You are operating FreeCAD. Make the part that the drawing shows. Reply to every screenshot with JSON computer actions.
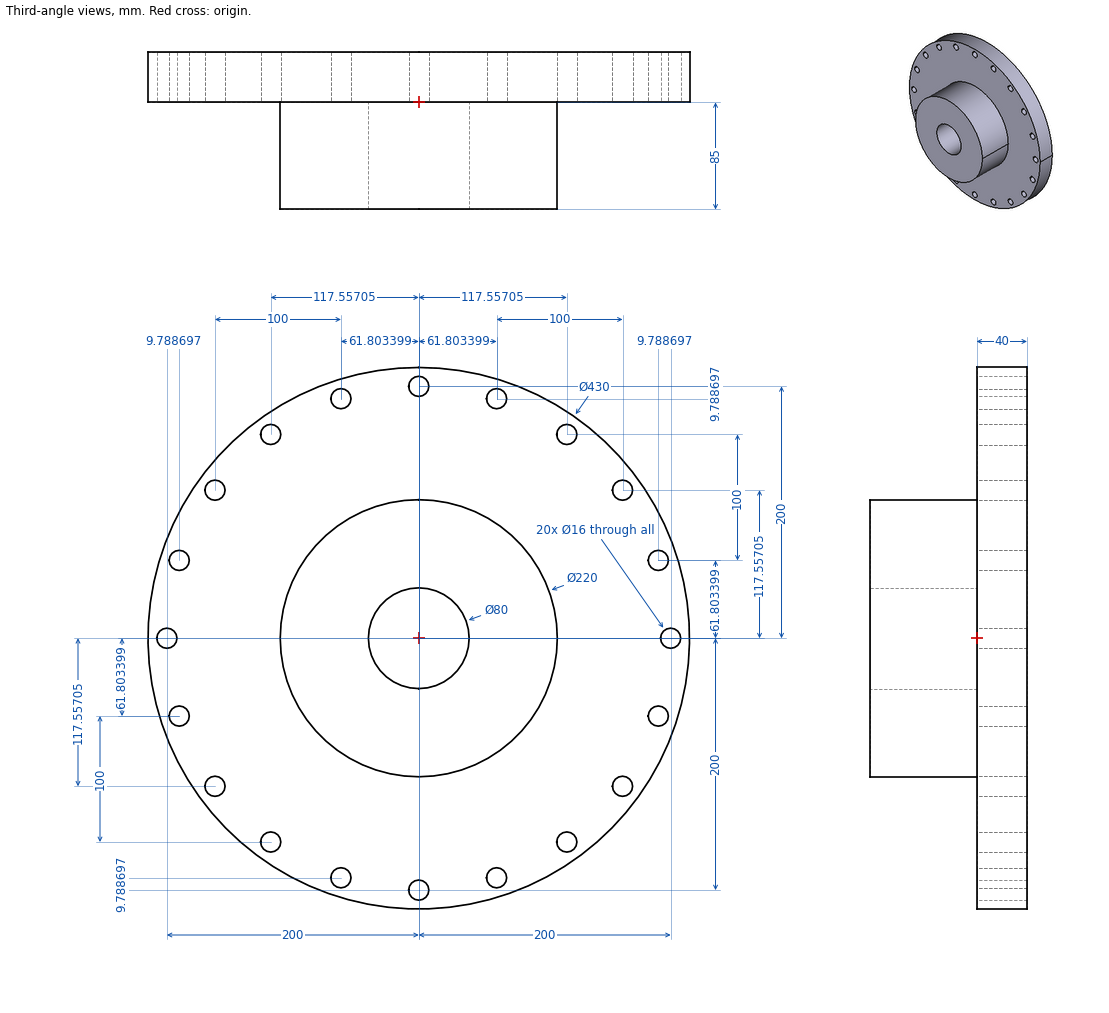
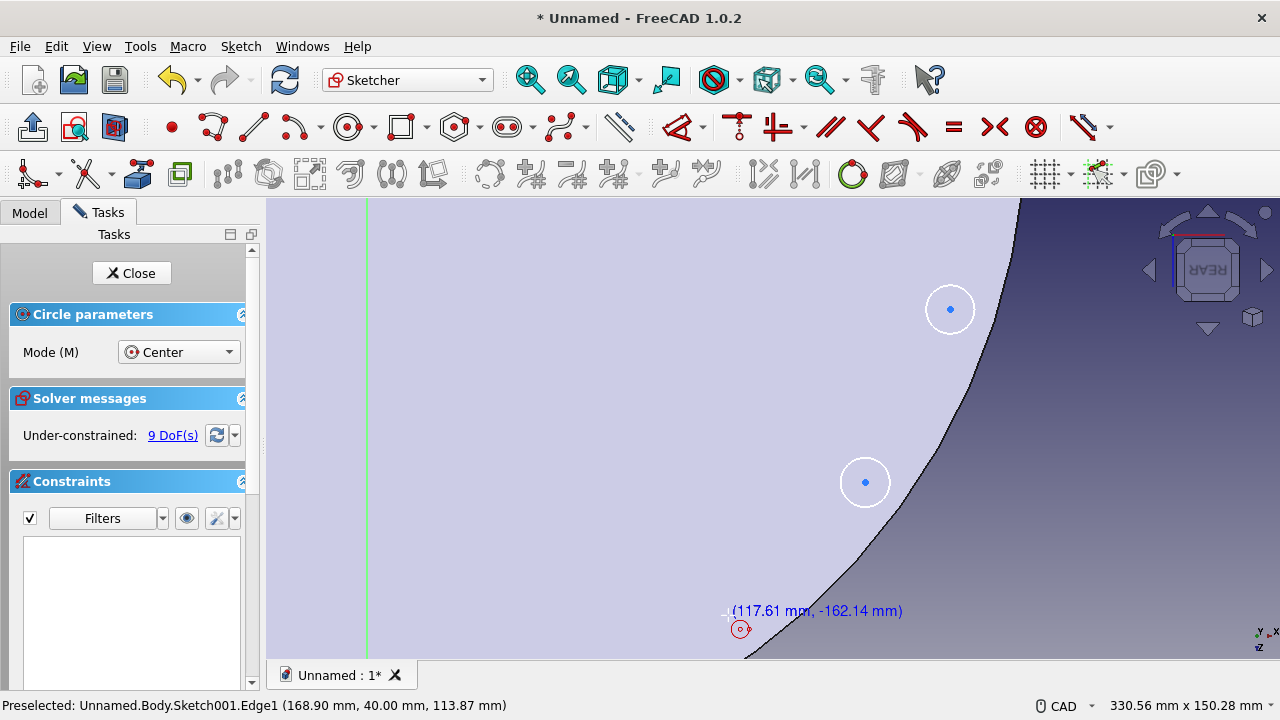
{"action": "scroll", "coordinate": [815, 530], "scroll_direction": "down", "scroll_amount": 7}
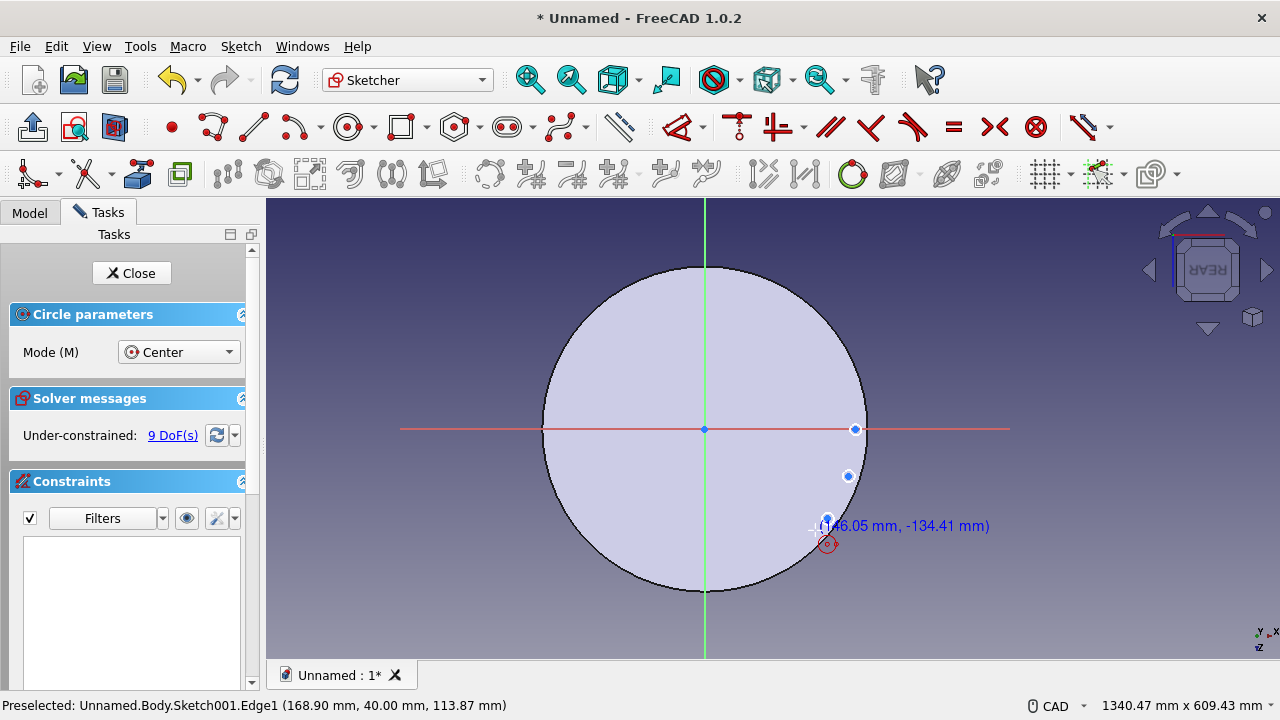
{"action": "left_click", "coordinate": [794, 552]}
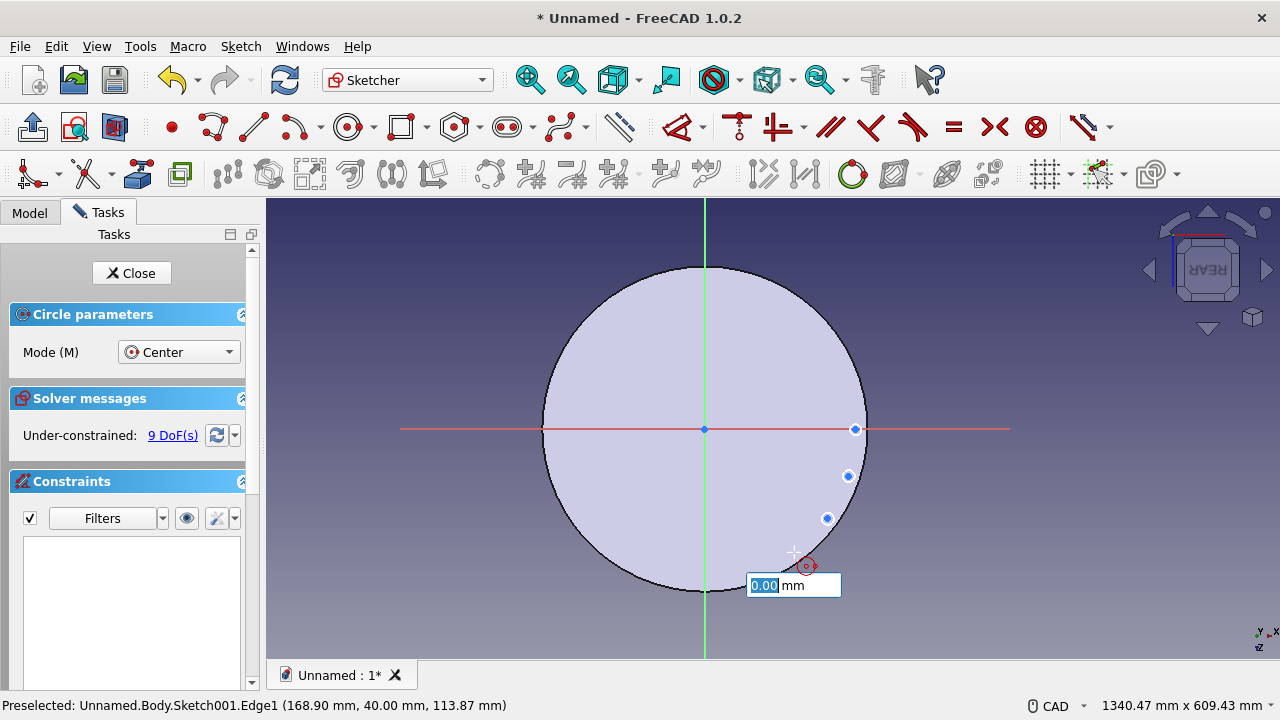
{"action": "scroll", "coordinate": [798, 547], "scroll_direction": "up", "scroll_amount": 5}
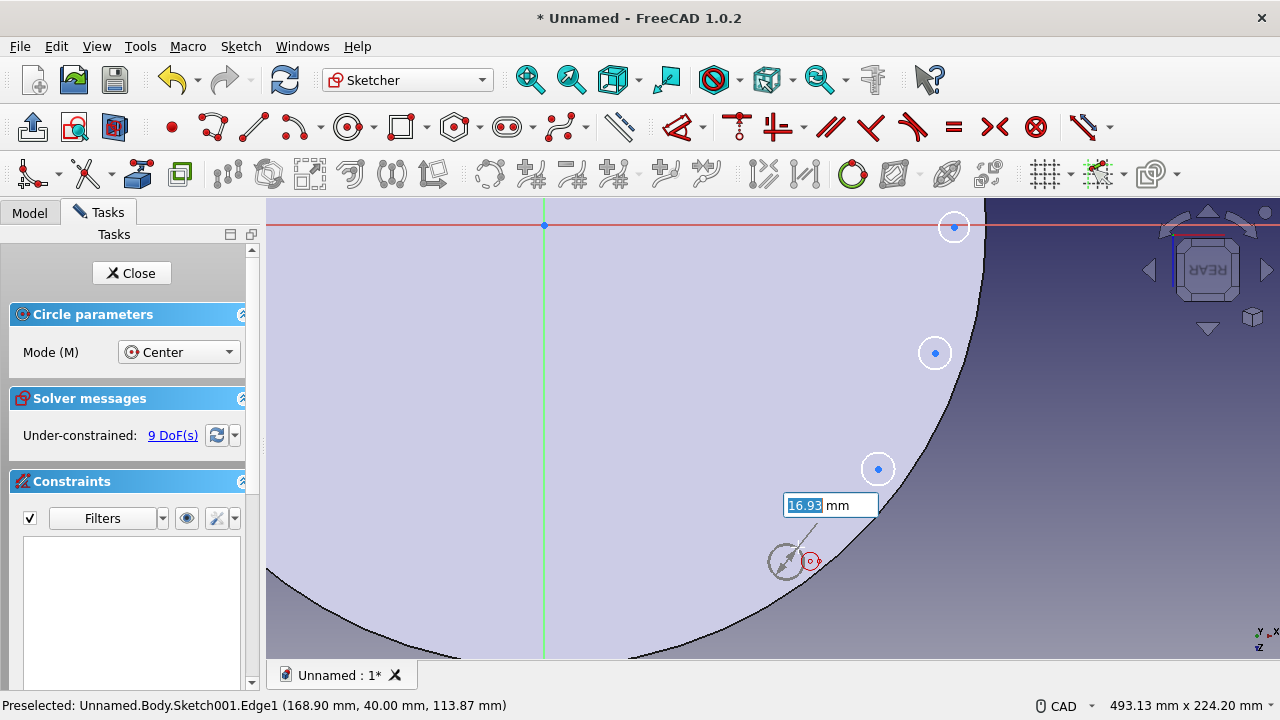
{"action": "left_click", "coordinate": [797, 546]}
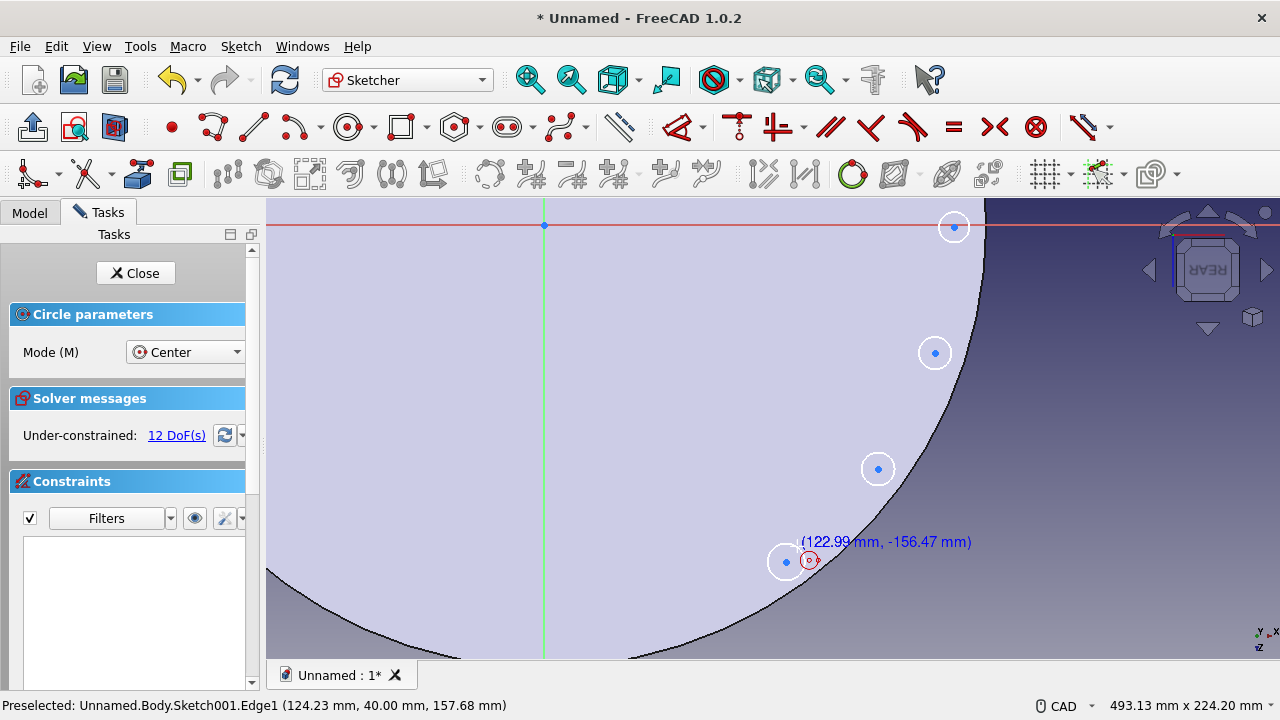
{"action": "scroll", "coordinate": [671, 616], "scroll_direction": "up", "scroll_amount": 2}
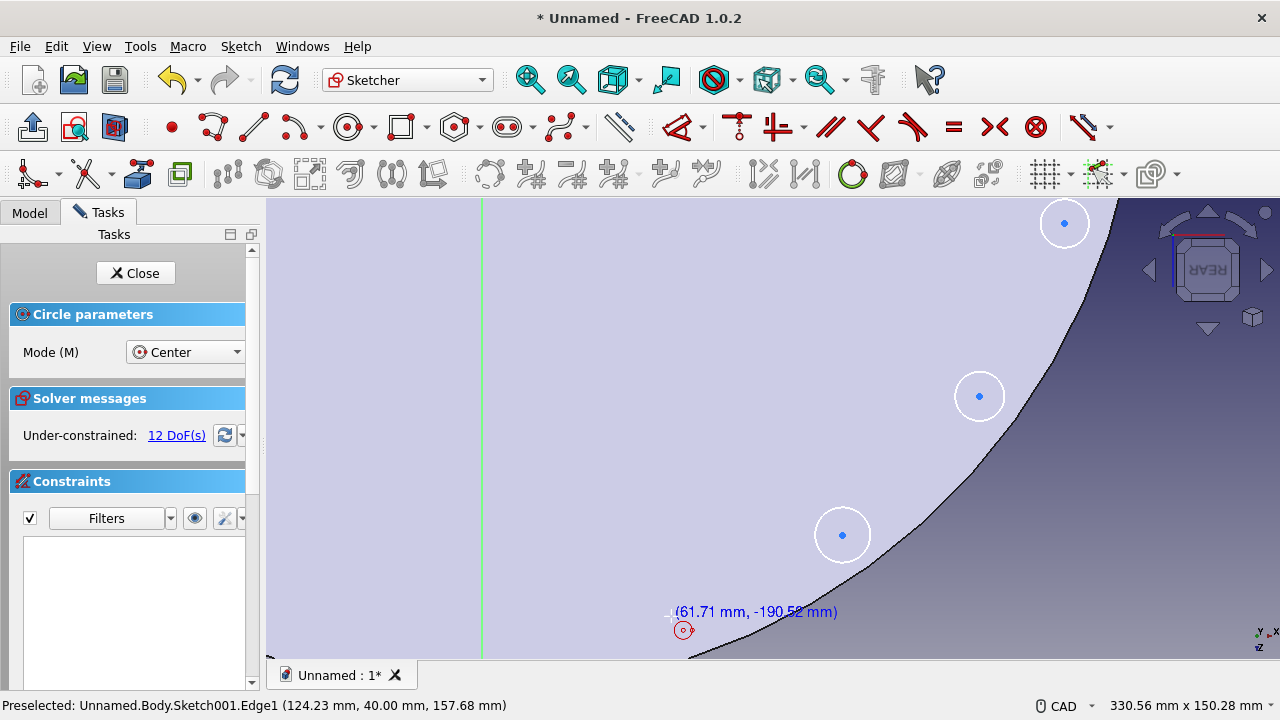
{"action": "scroll", "coordinate": [777, 558], "scroll_direction": "down", "scroll_amount": 7}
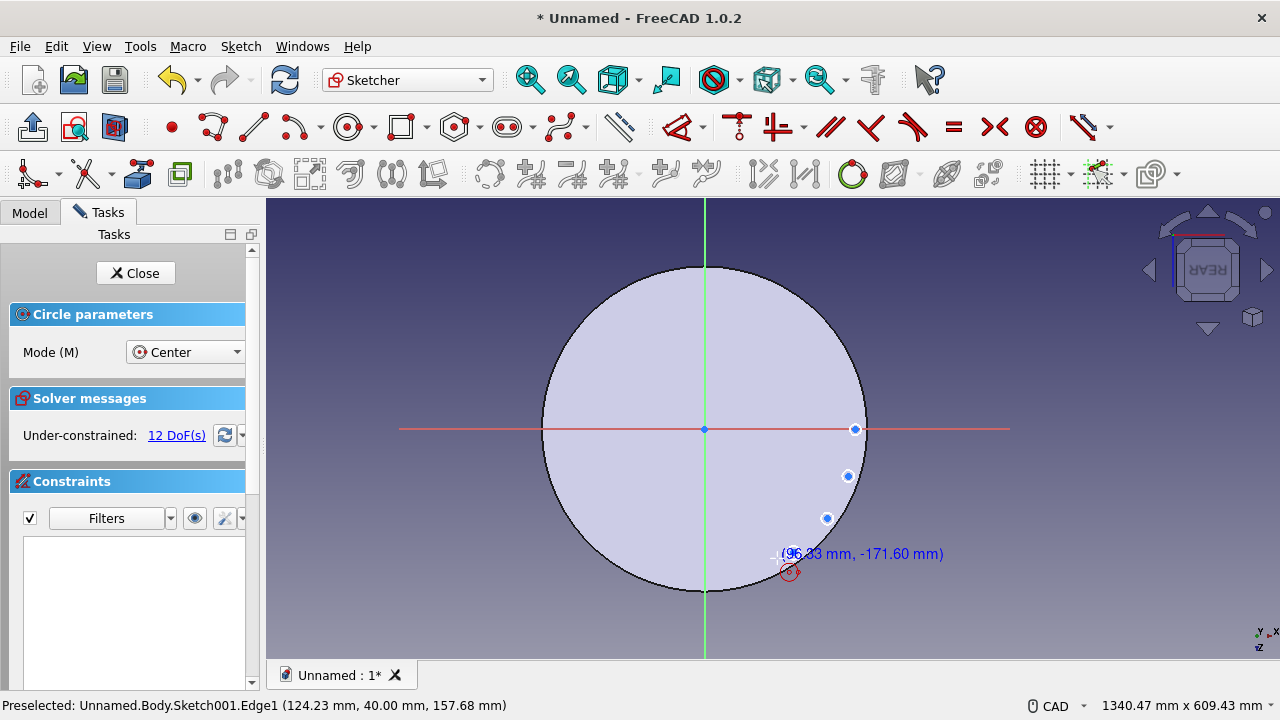
{"action": "left_click", "coordinate": [751, 573]}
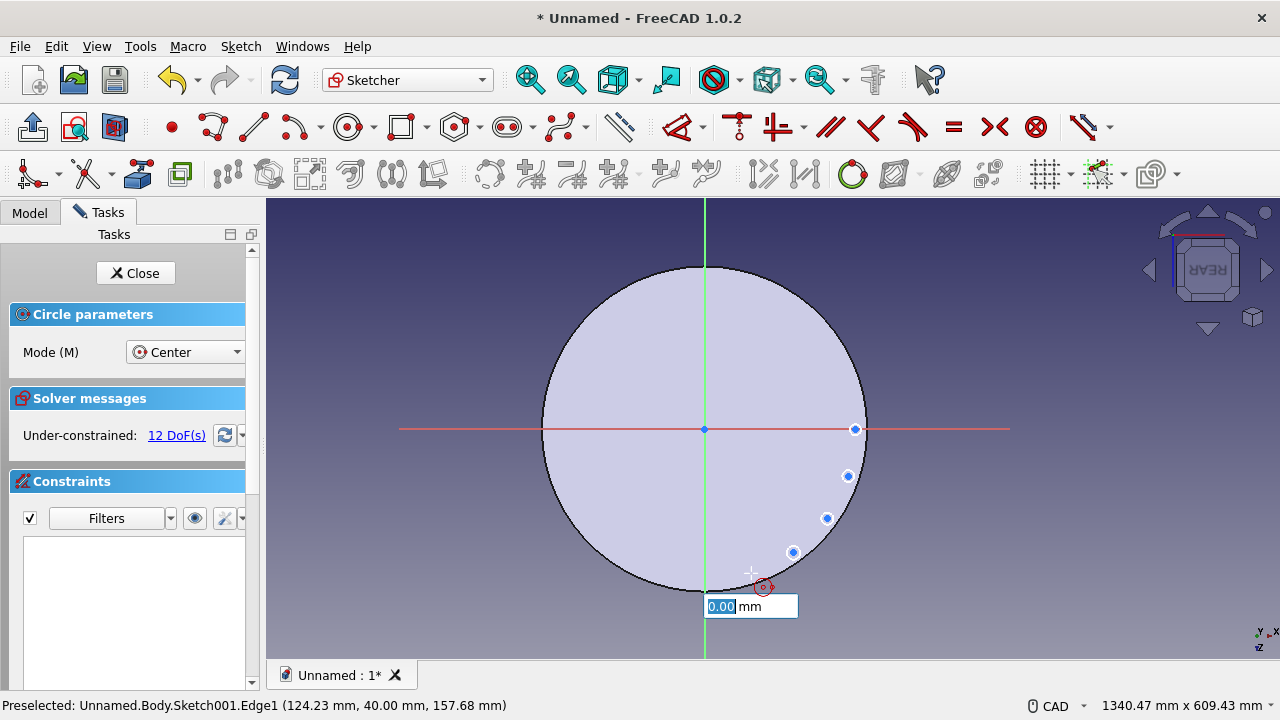
{"action": "scroll", "coordinate": [756, 569], "scroll_direction": "up", "scroll_amount": 5}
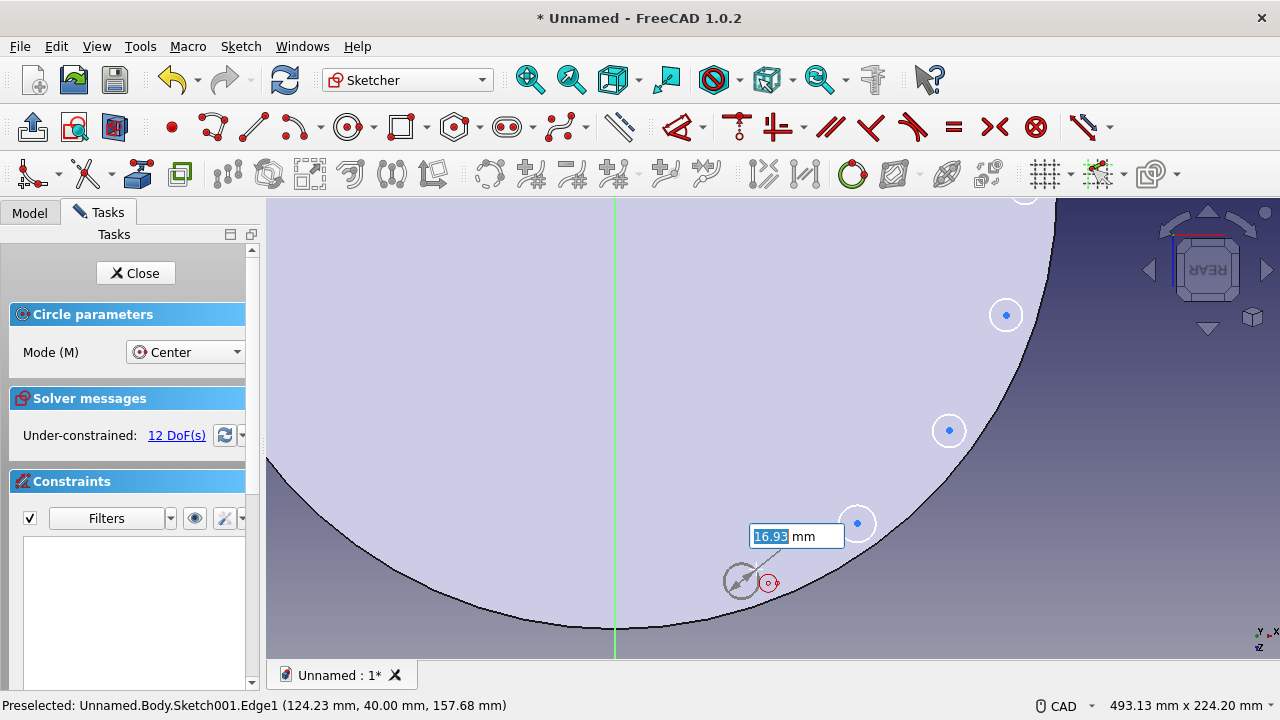
{"action": "left_click", "coordinate": [754, 567]}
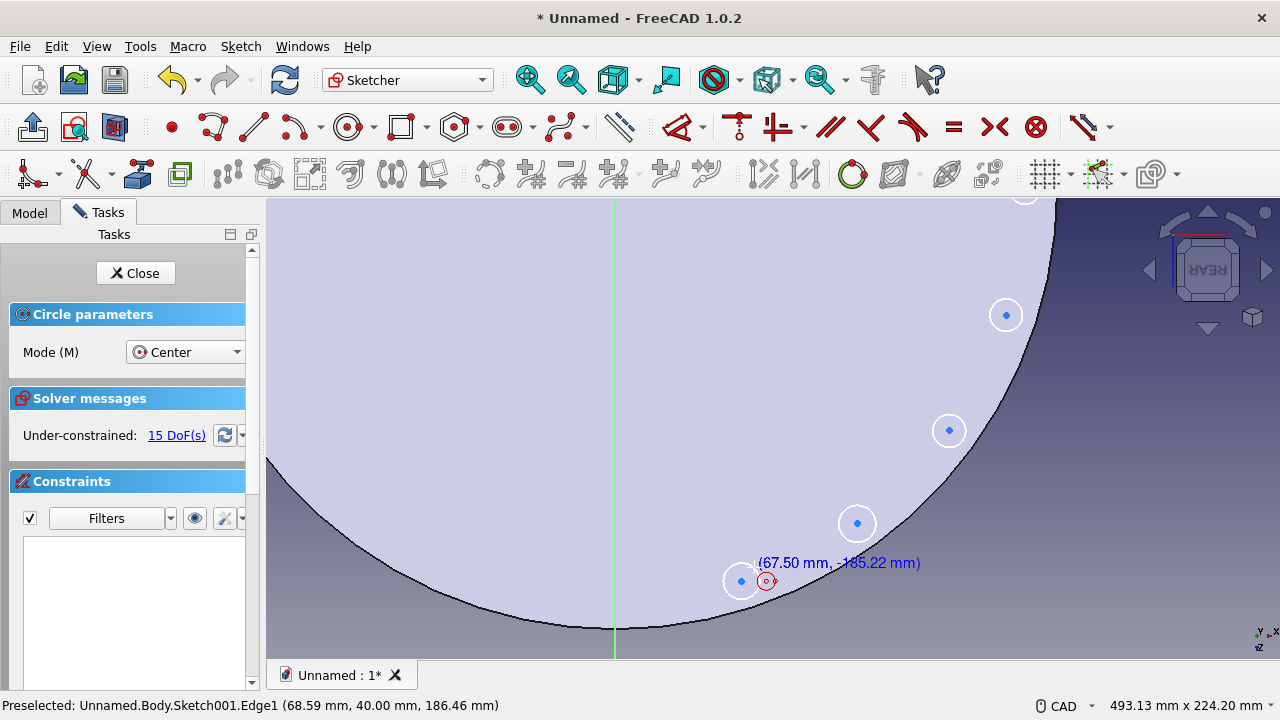
{"action": "scroll", "coordinate": [615, 598], "scroll_direction": "up", "scroll_amount": 2}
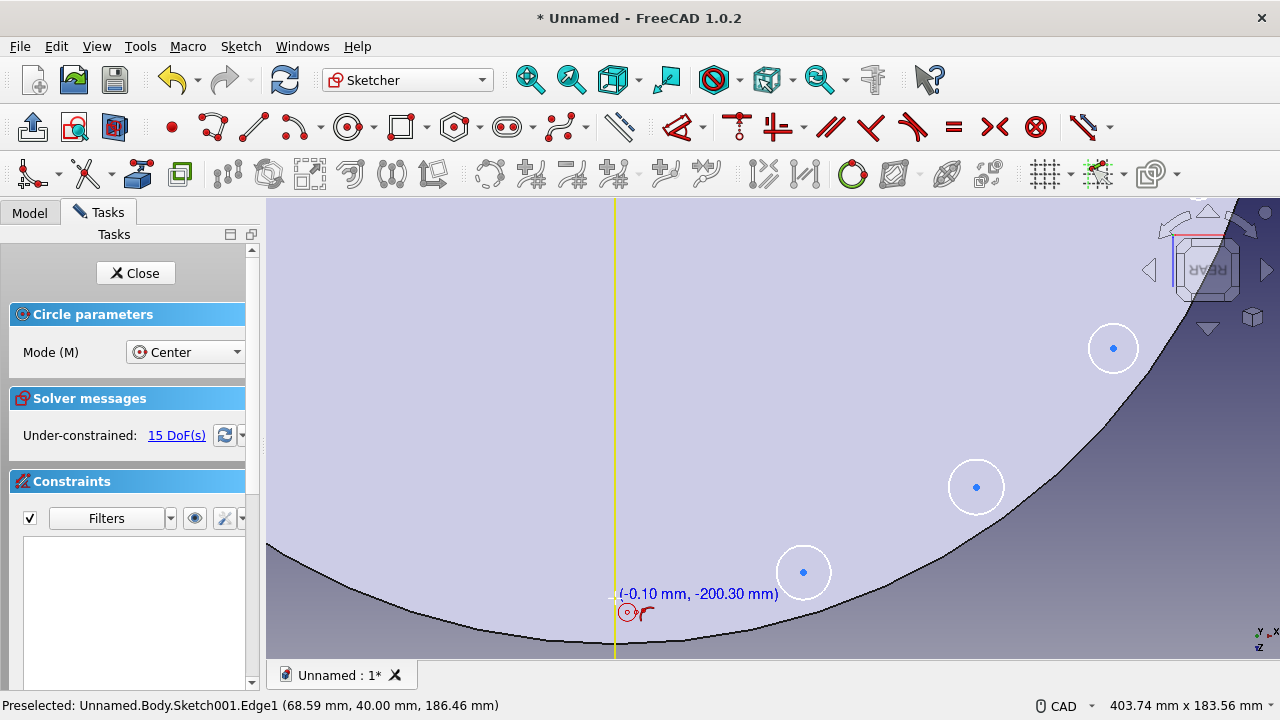
{"action": "scroll", "coordinate": [734, 574], "scroll_direction": "down", "scroll_amount": 7}